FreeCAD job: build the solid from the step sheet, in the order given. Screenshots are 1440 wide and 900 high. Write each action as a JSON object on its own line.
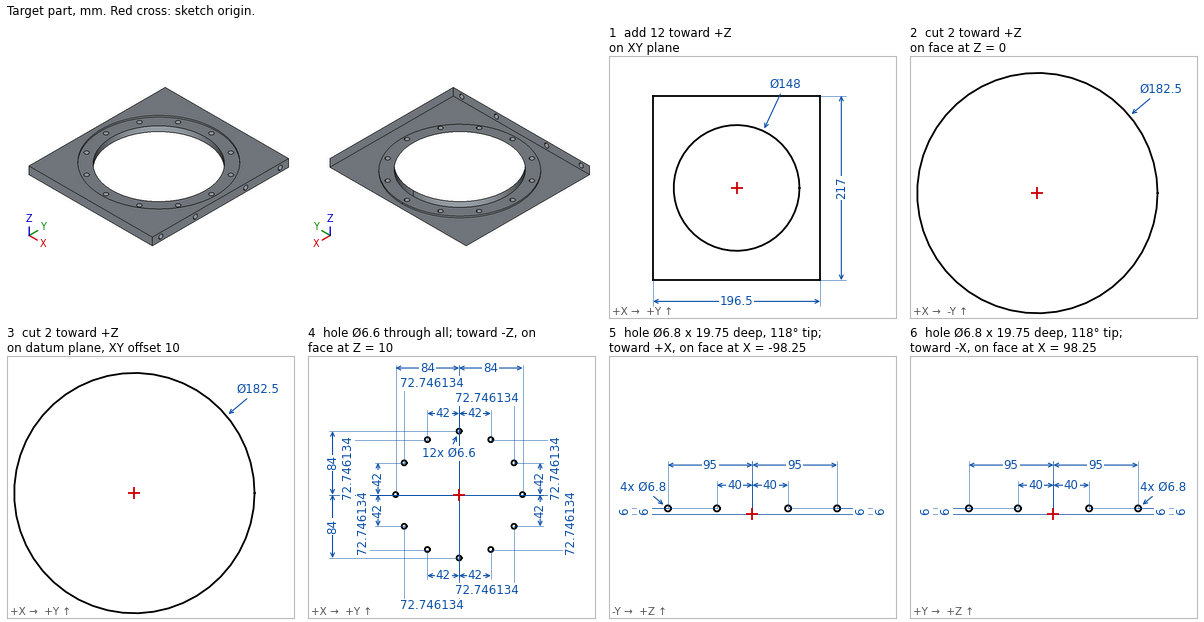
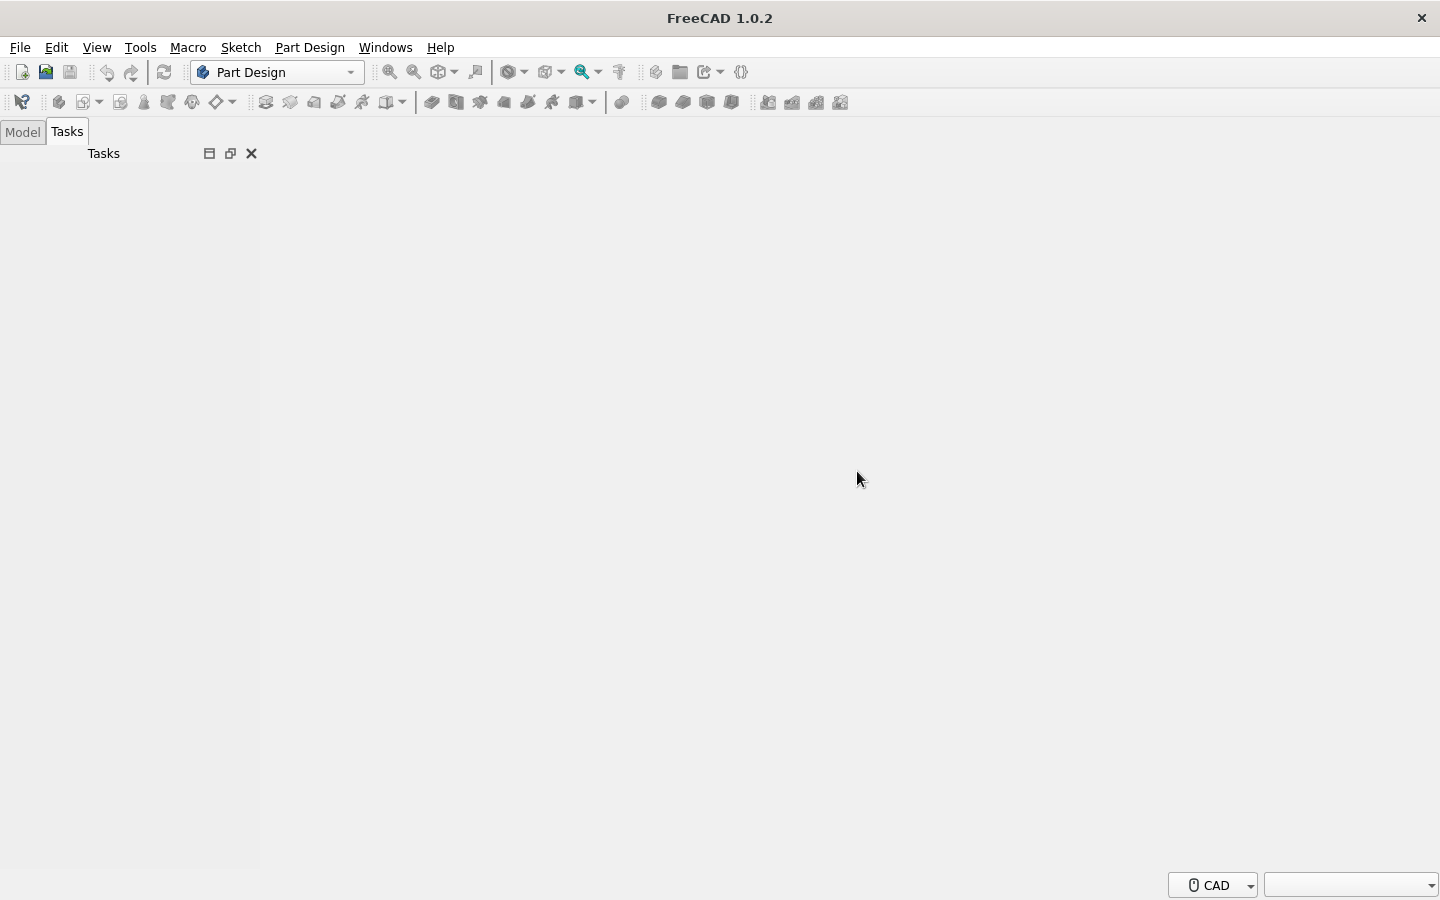
{"action": "left_click", "coordinate": [22, 72]}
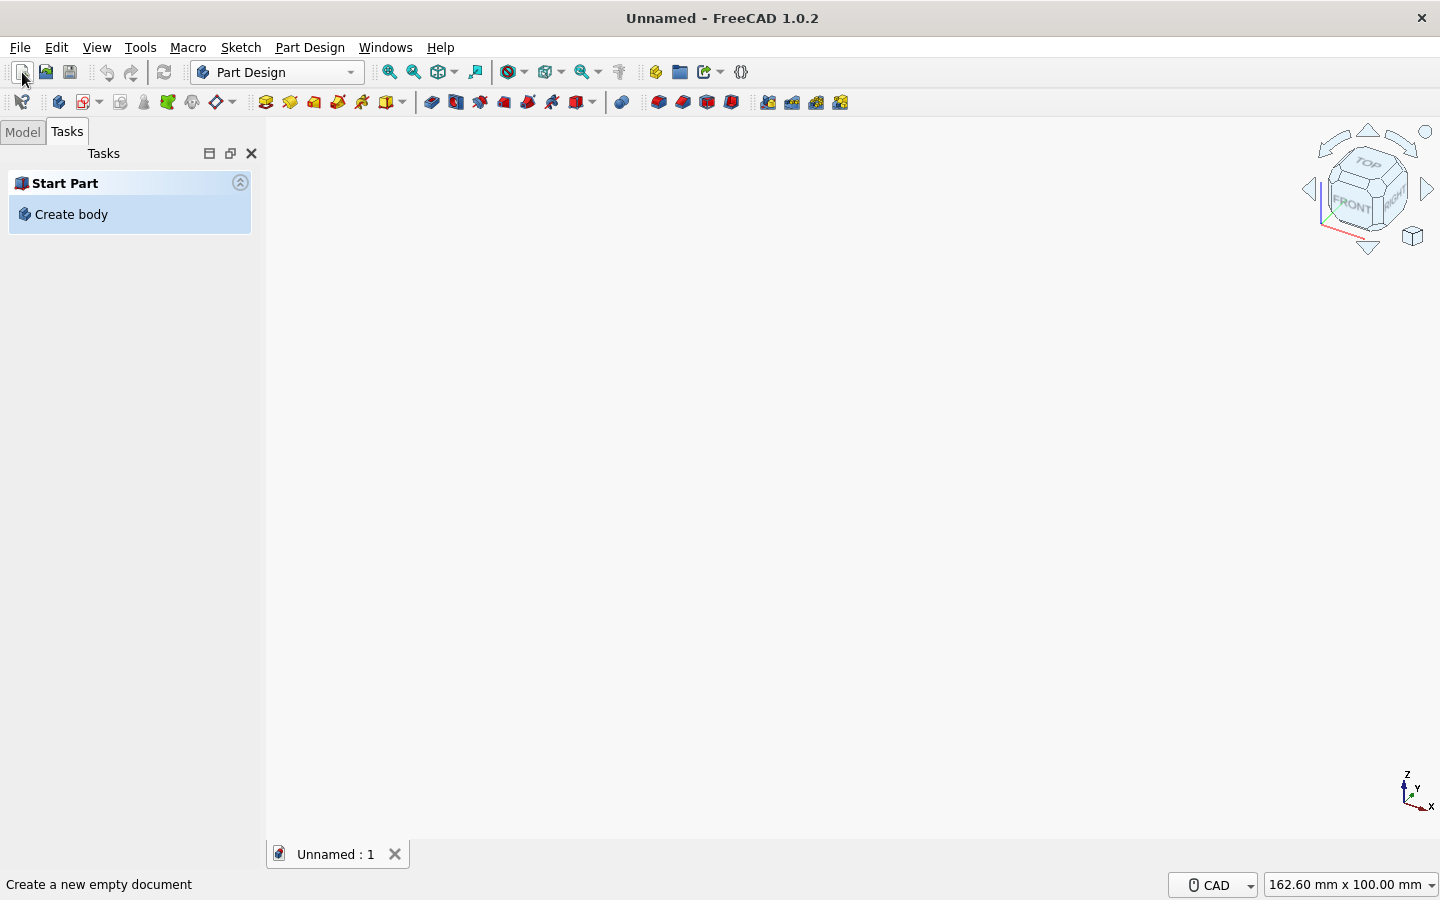
{"action": "left_click", "coordinate": [84, 102]}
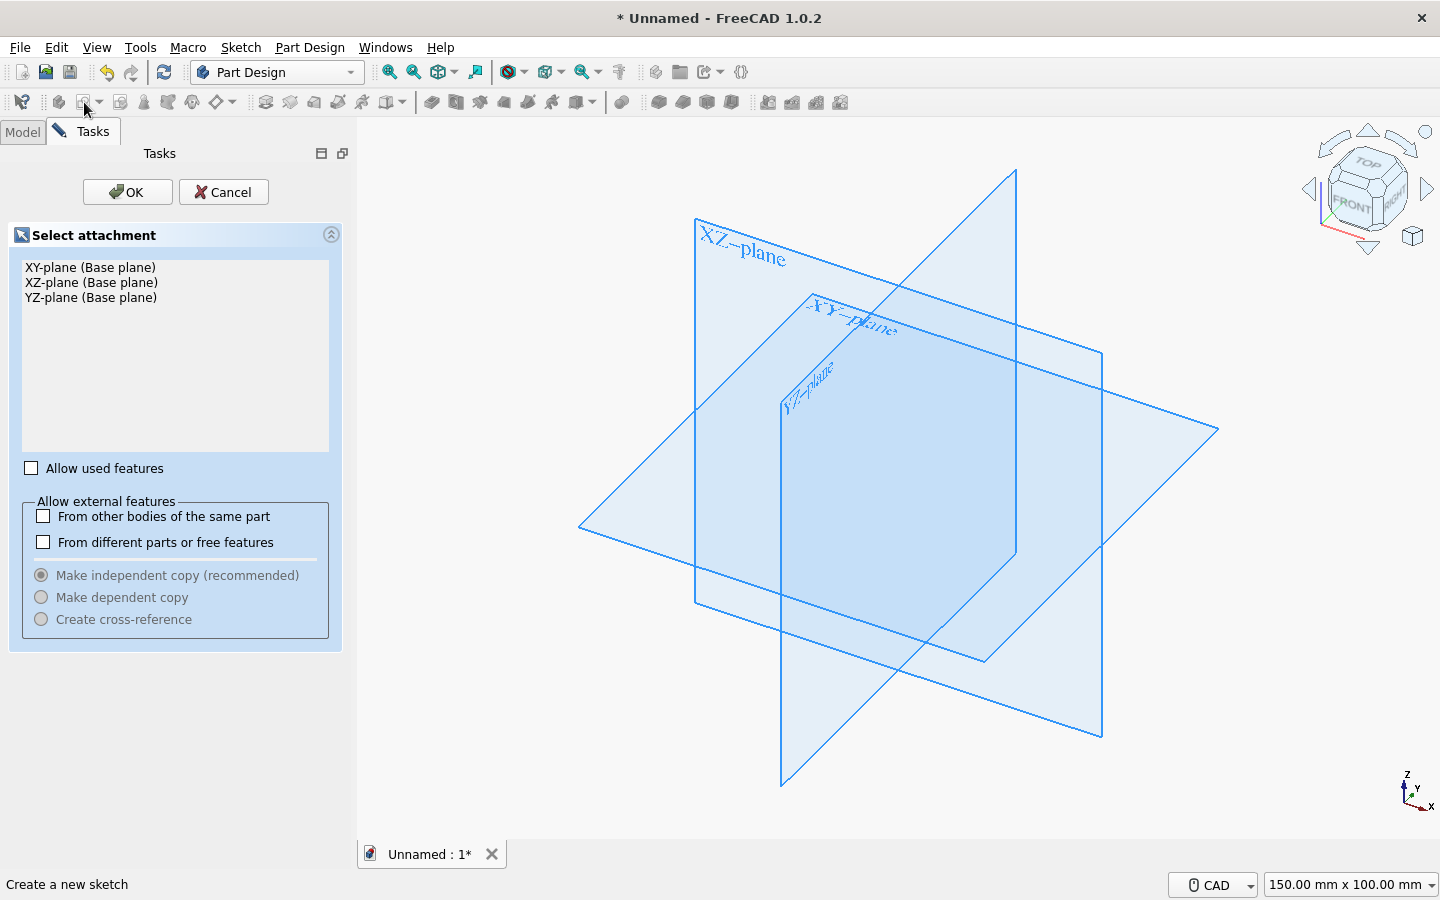
{"action": "left_click", "coordinate": [82, 268]}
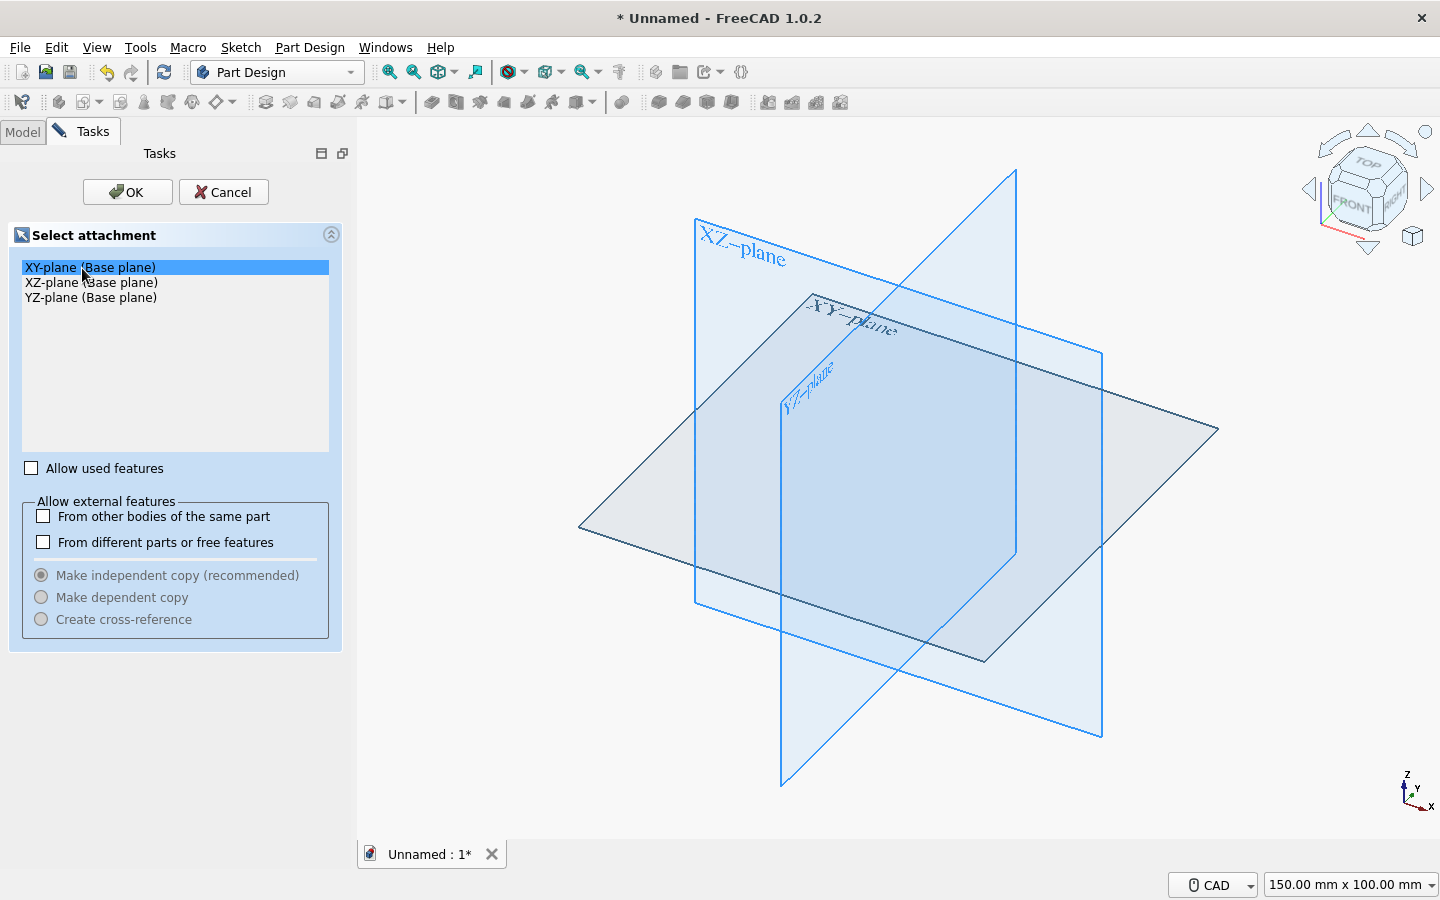
{"action": "left_click", "coordinate": [128, 192]}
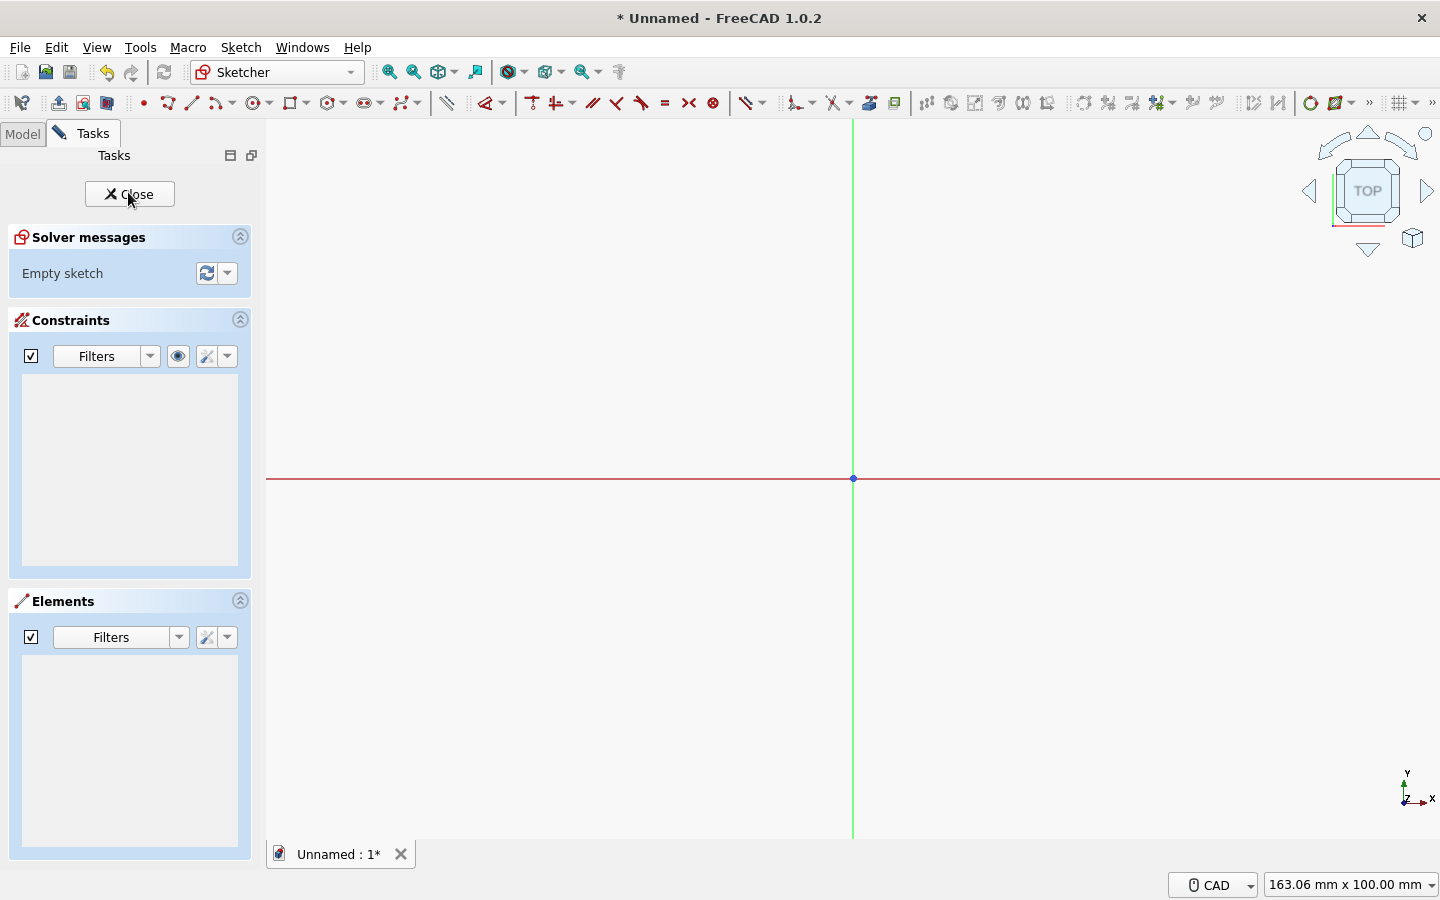
{"action": "scroll", "coordinate": [755, 479], "scroll_direction": "down", "scroll_amount": 6}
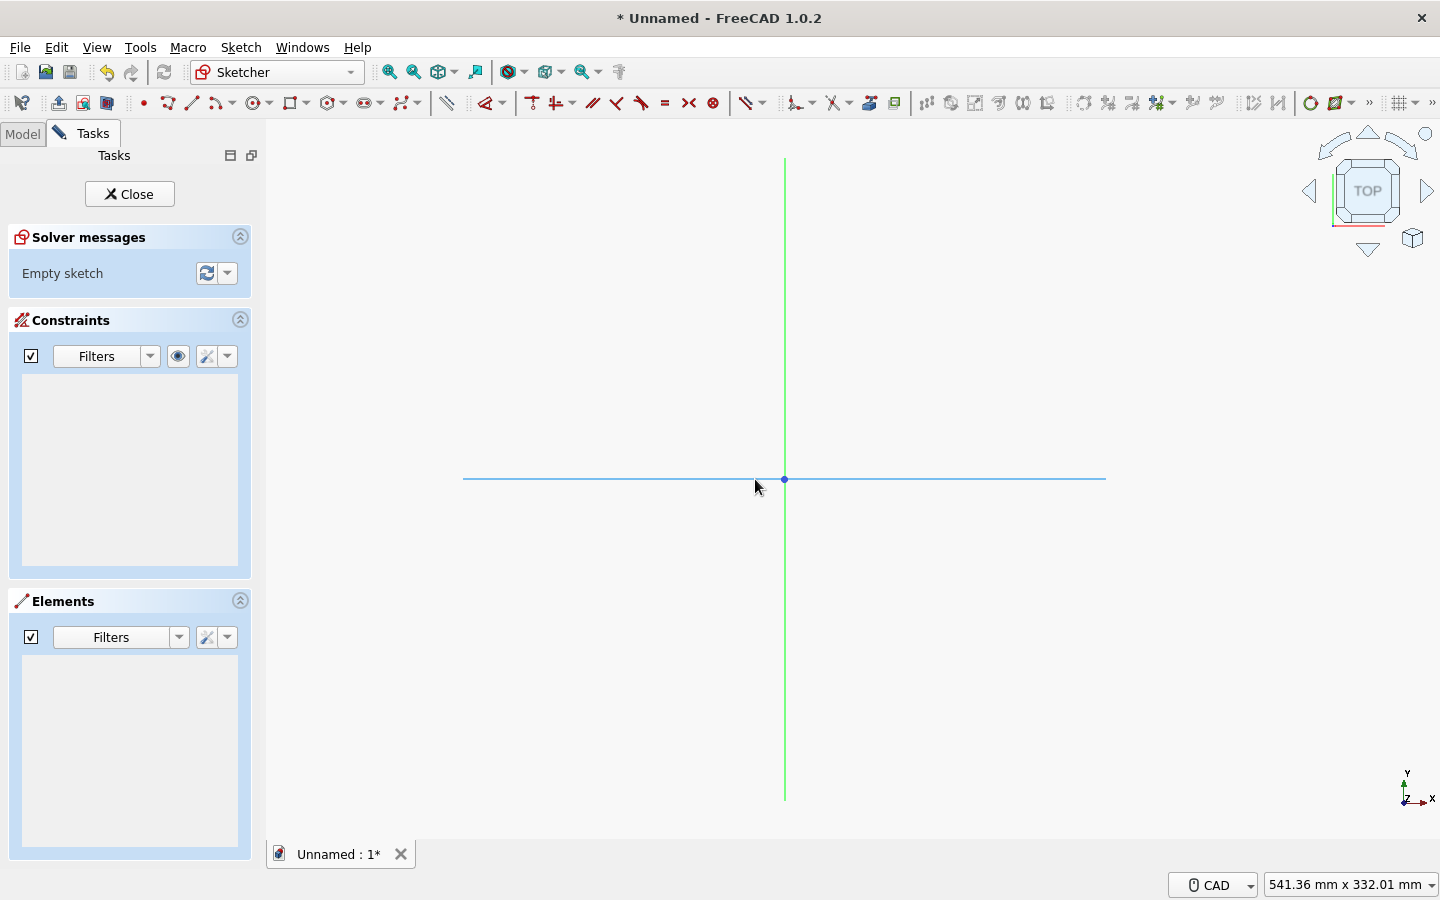
{"action": "key", "text": "g v"}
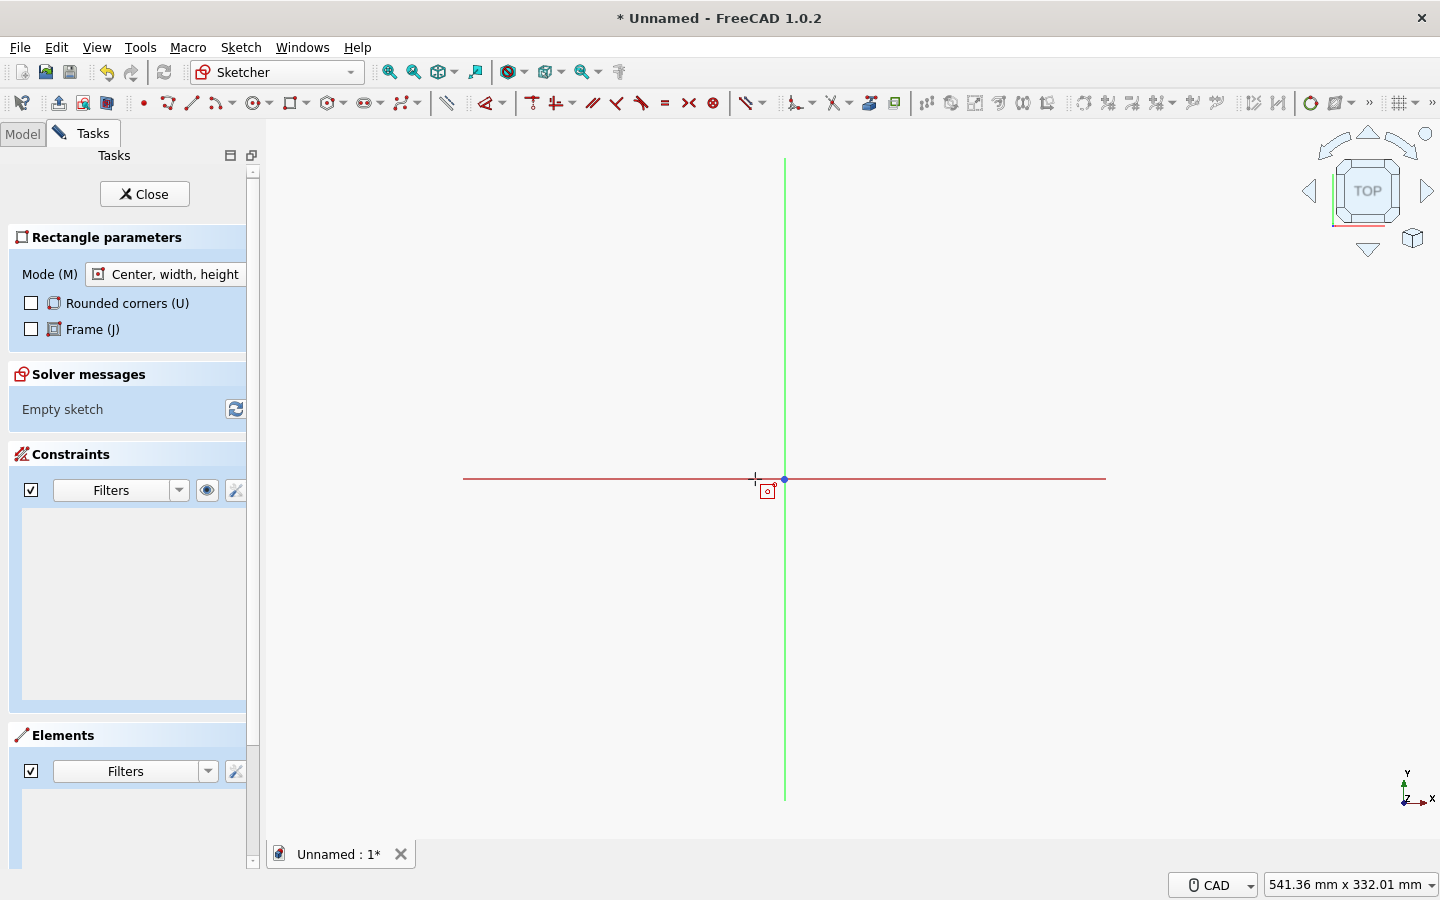
{"action": "left_click", "coordinate": [785, 479]}
{"action": "mouse_move", "coordinate": [998, 244]}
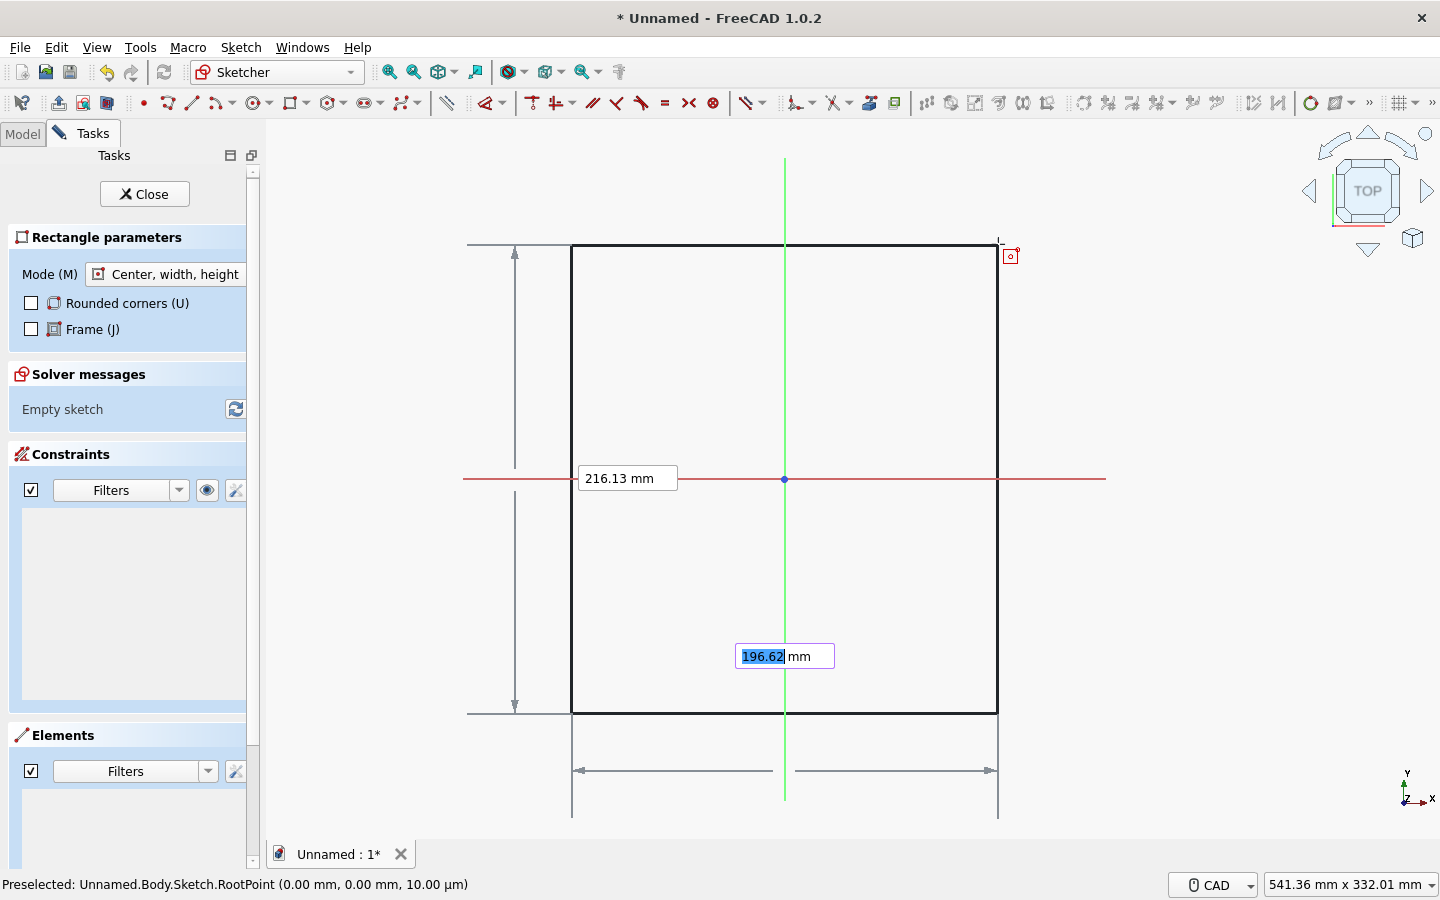
{"action": "type", "text": "196.5"}
{"action": "key", "text": "Tab"}
{"action": "type", "text": "217"}
{"action": "key", "text": "Return"}